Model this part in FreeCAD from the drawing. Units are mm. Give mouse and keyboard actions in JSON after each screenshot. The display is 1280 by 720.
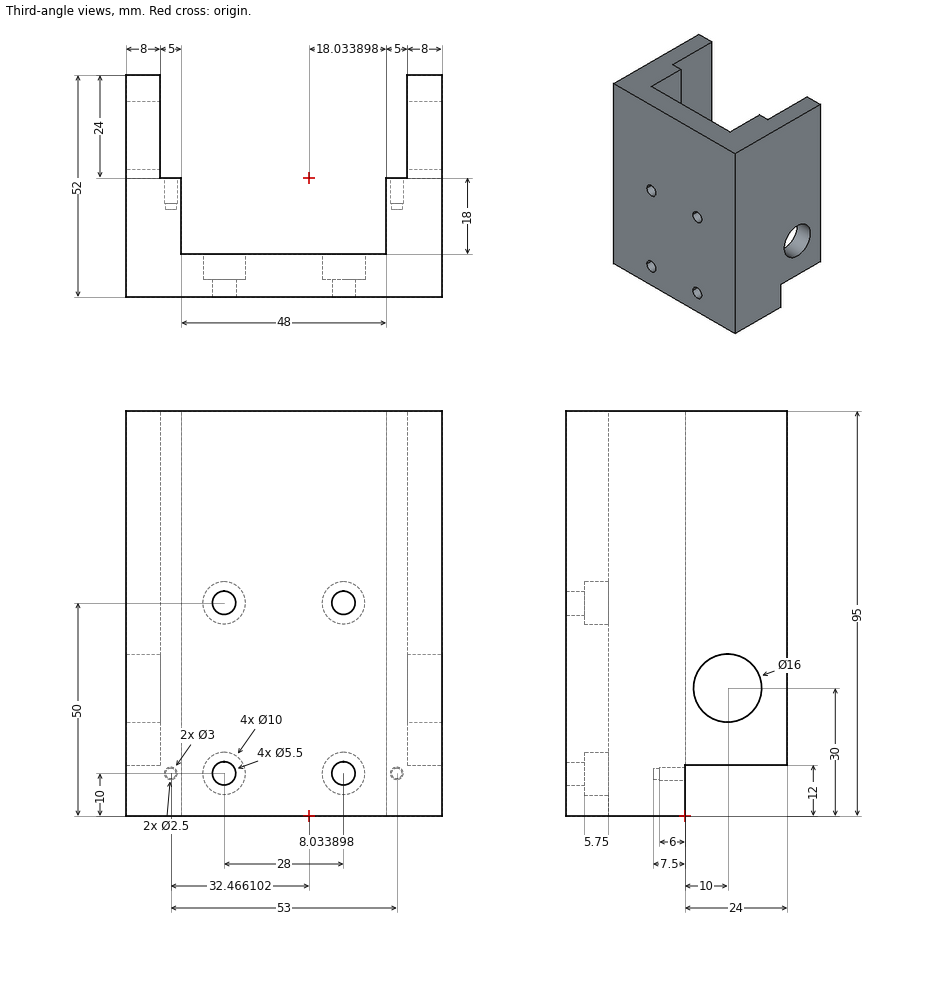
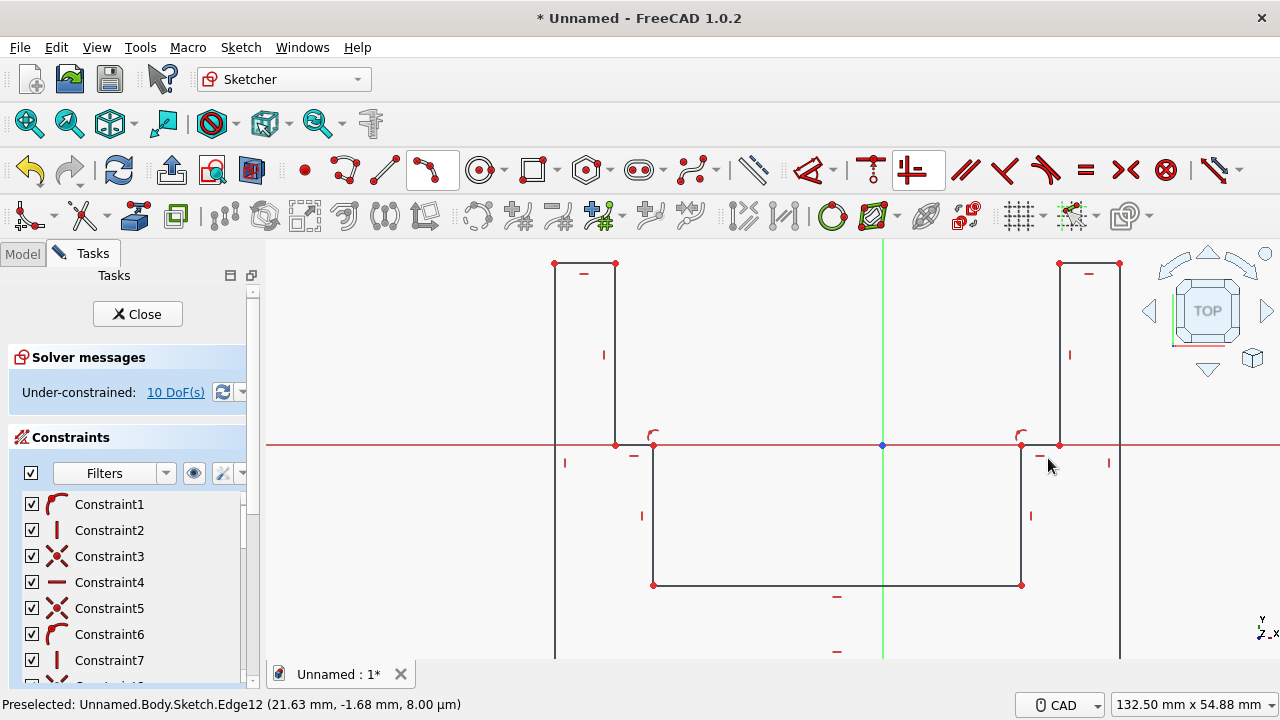
{"action": "left_click", "coordinate": [642, 445]}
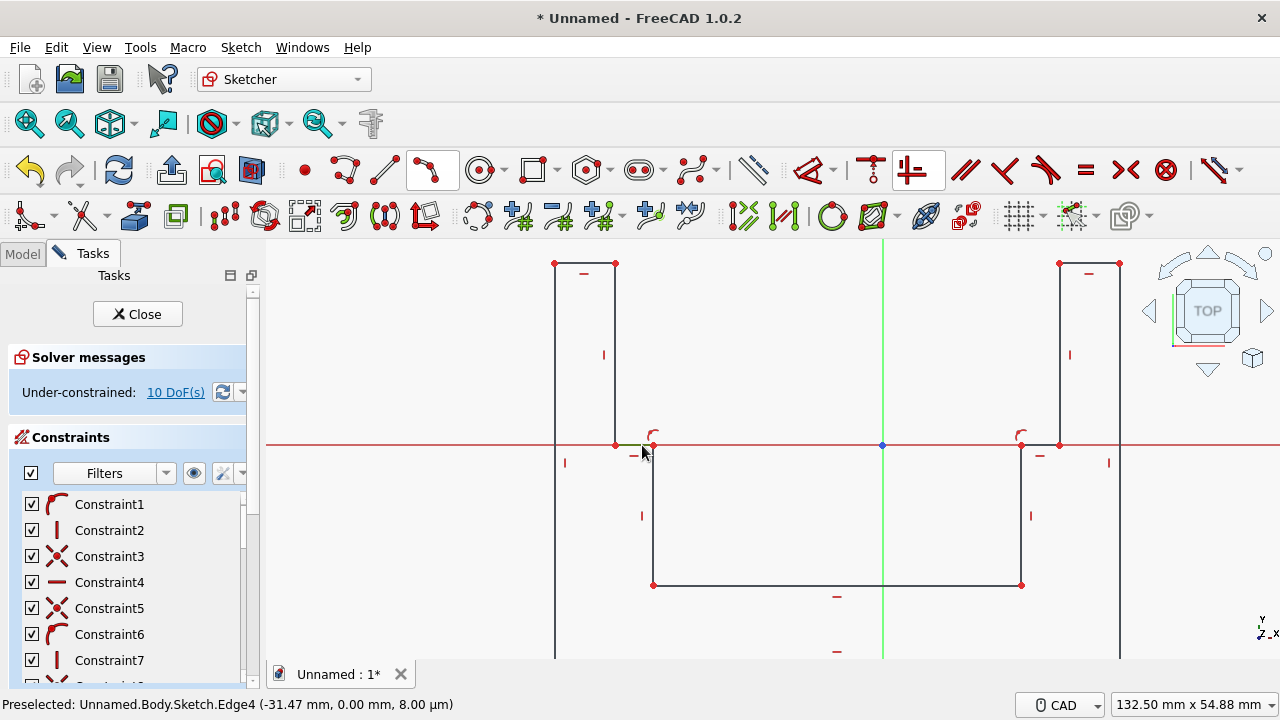
{"action": "left_click", "coordinate": [836, 170]}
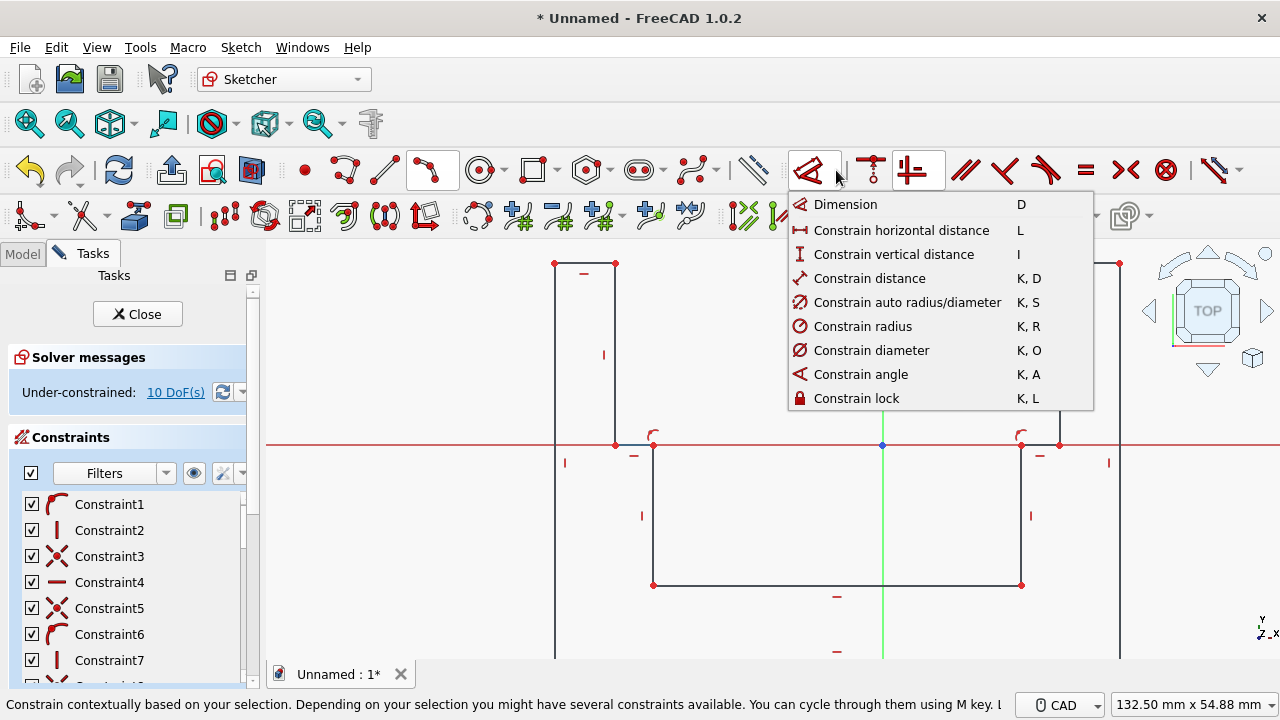
{"action": "left_click", "coordinate": [941, 230]}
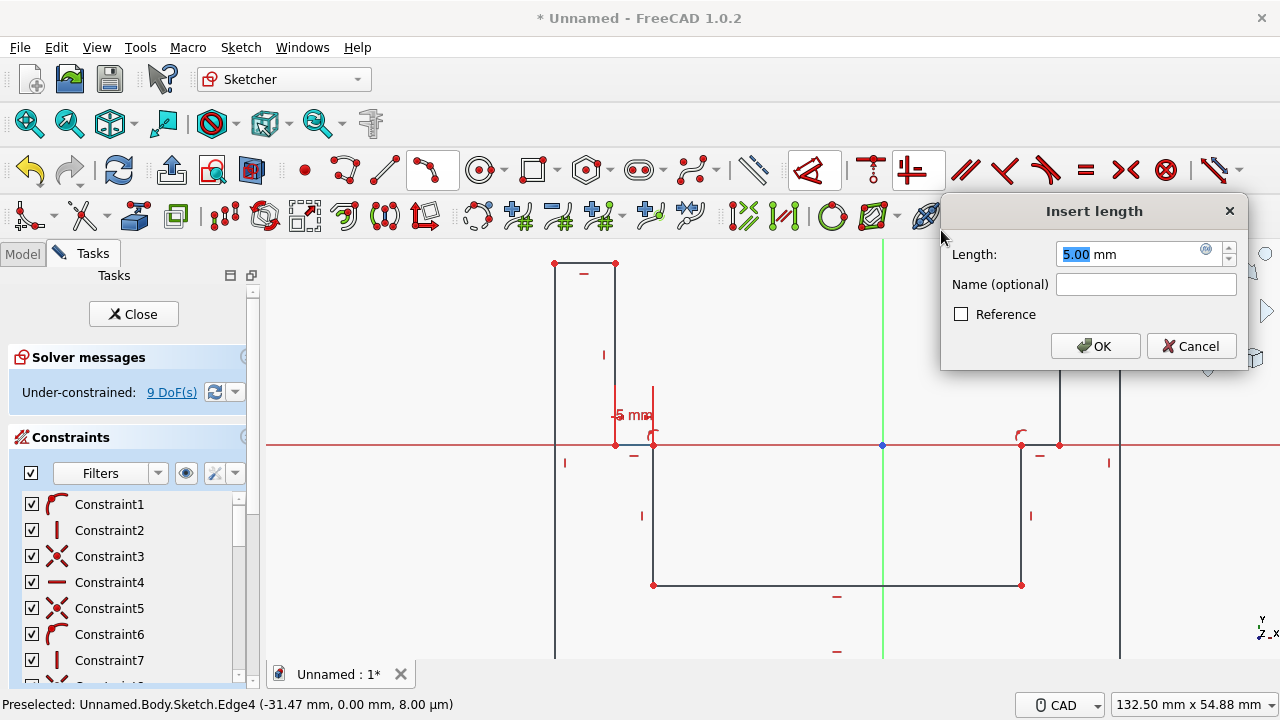
{"action": "type", "text": "5"}
{"action": "key", "text": "Return"}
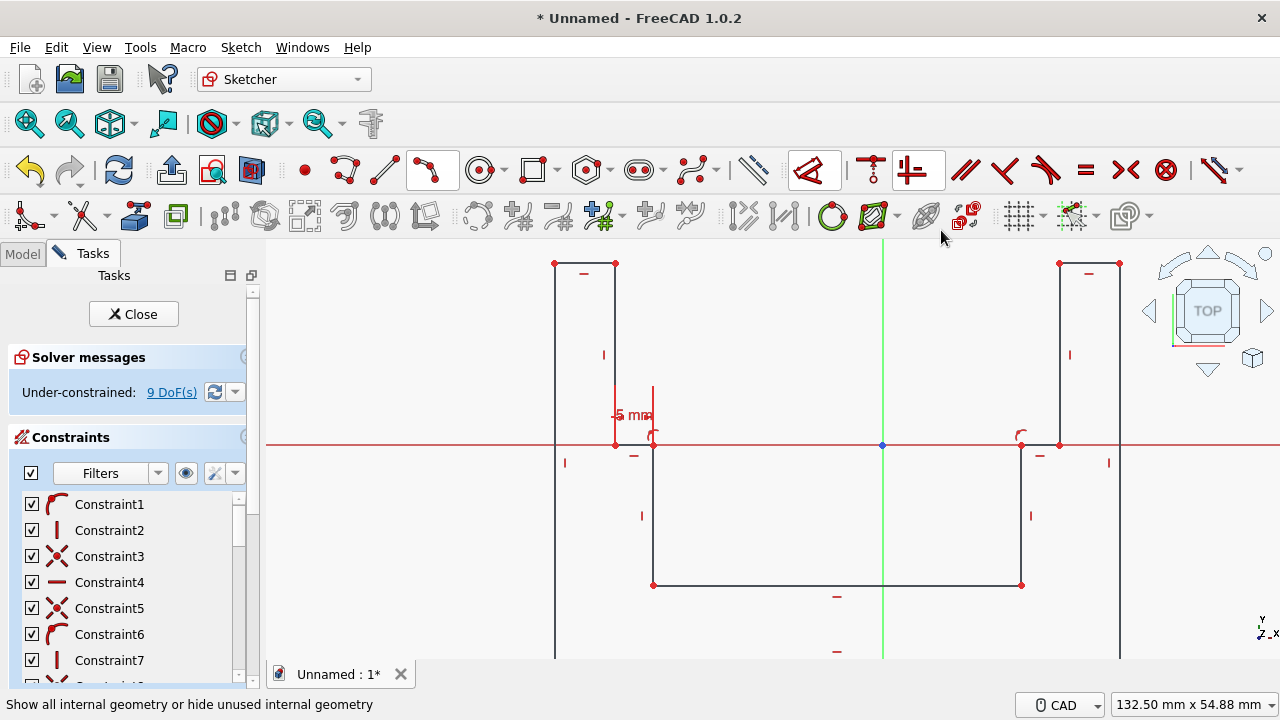
{"action": "scroll", "coordinate": [435, 425], "scroll_direction": "down", "scroll_amount": 2}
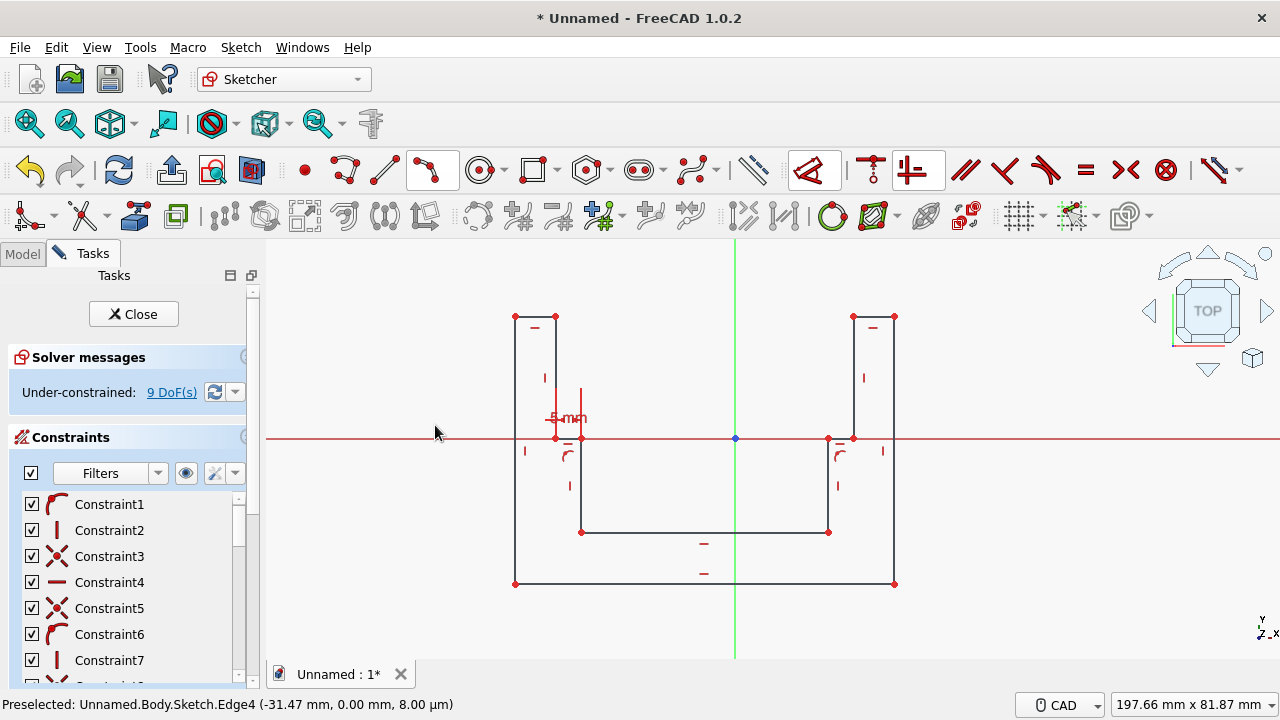
{"action": "left_click", "coordinate": [544, 317]}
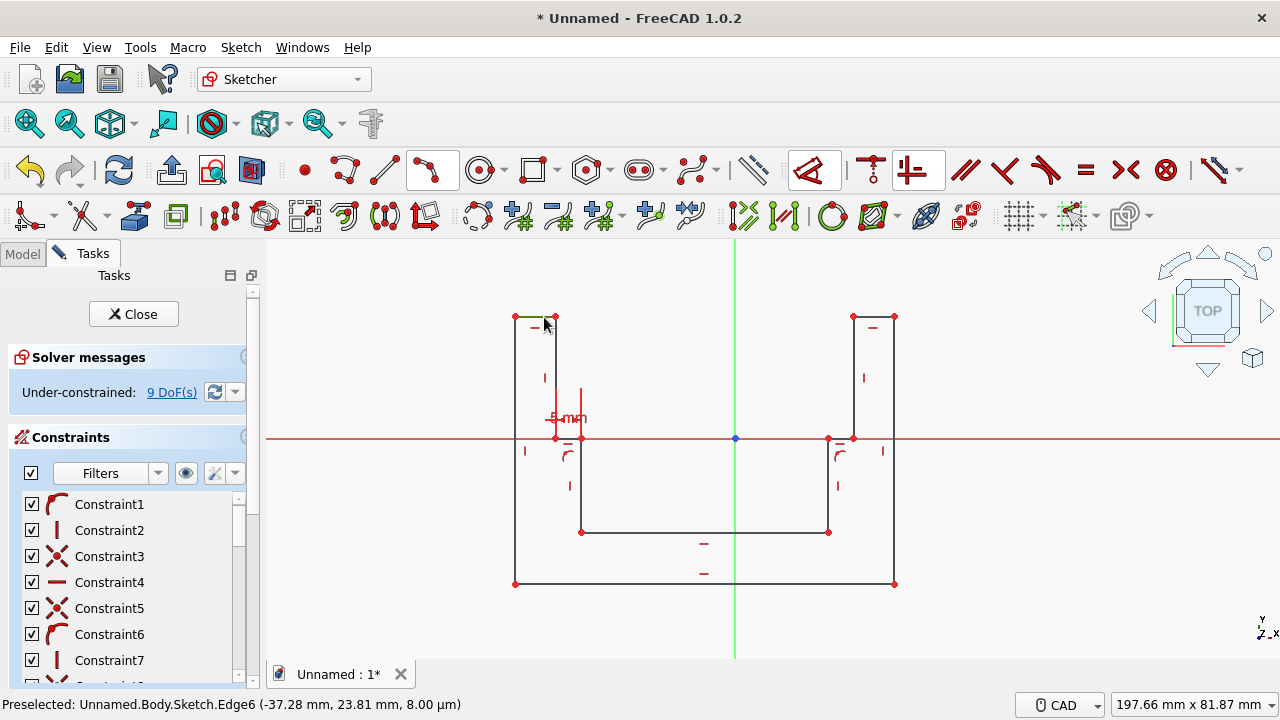
{"action": "key", "text": "l"}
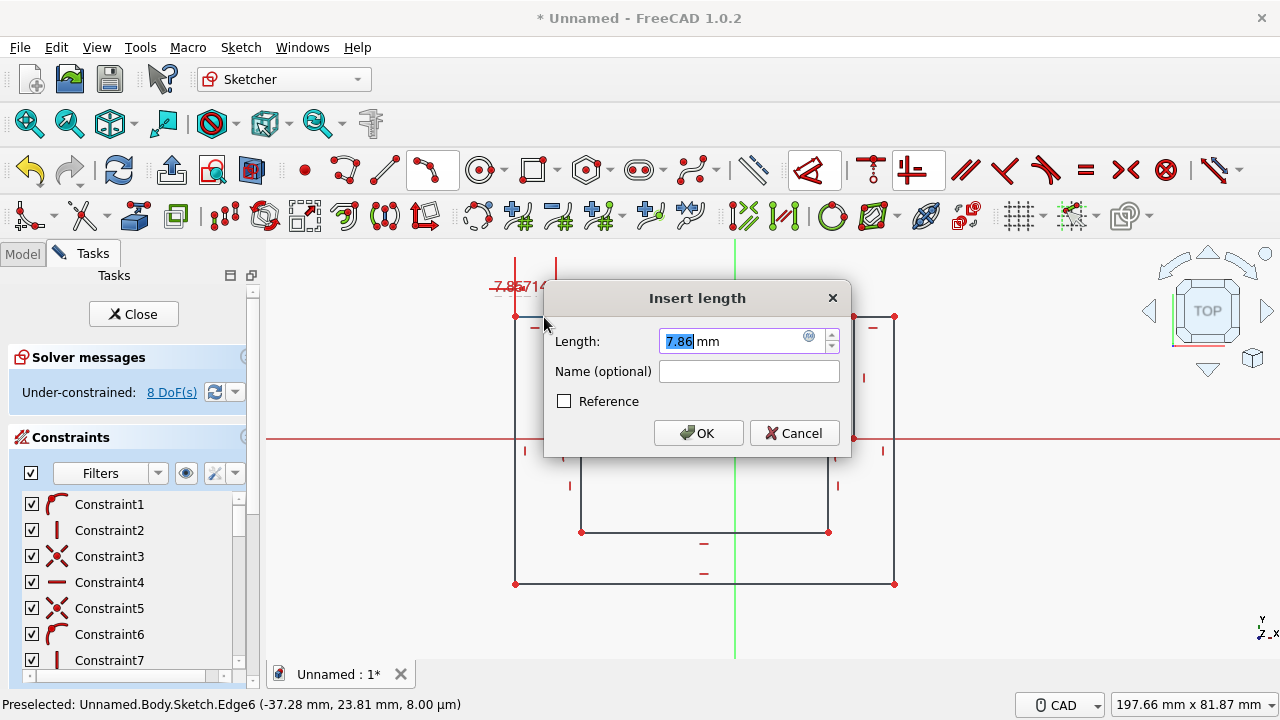
{"action": "type", "text": "8"}
{"action": "key", "text": "Return"}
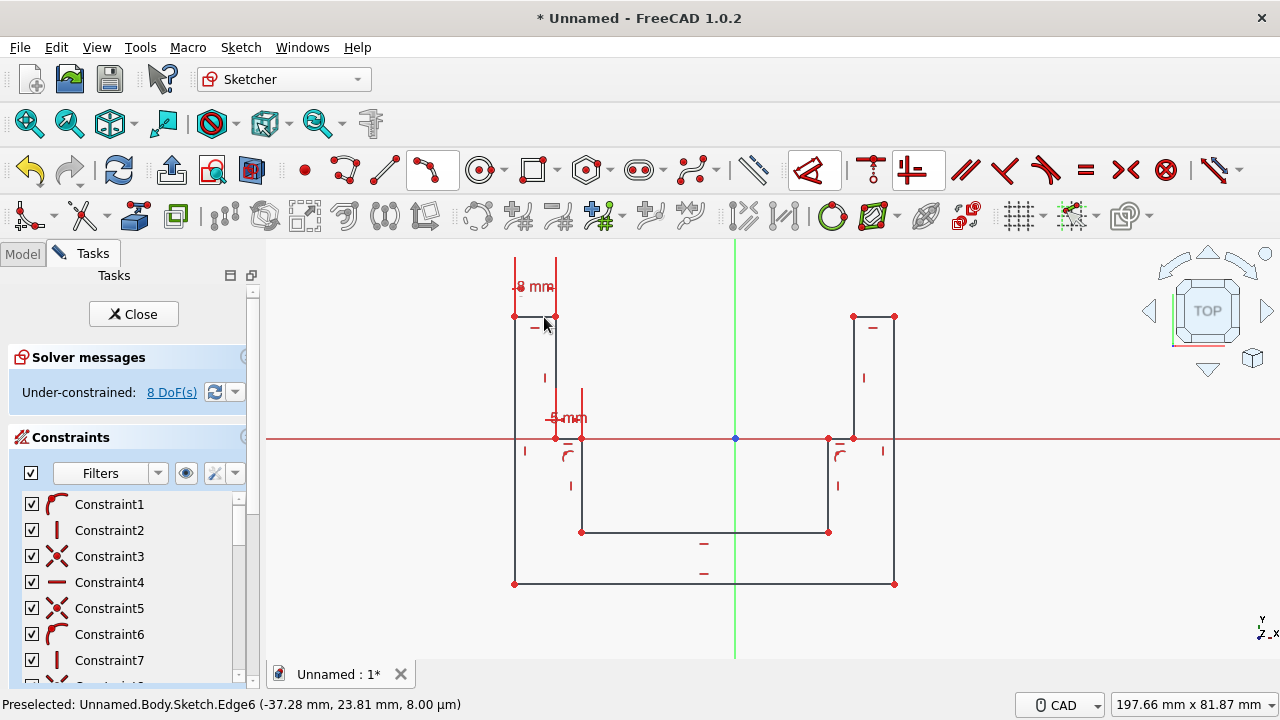
{"action": "left_click", "coordinate": [882, 317]}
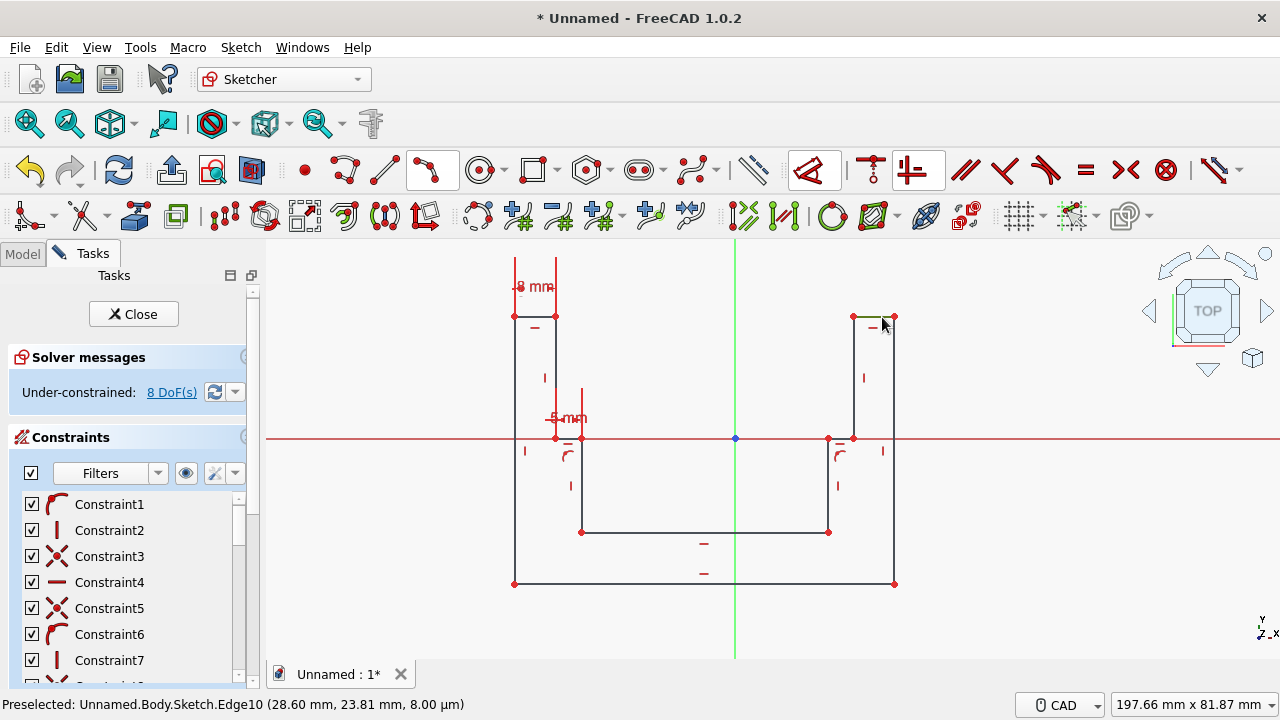
{"action": "key", "text": "l"}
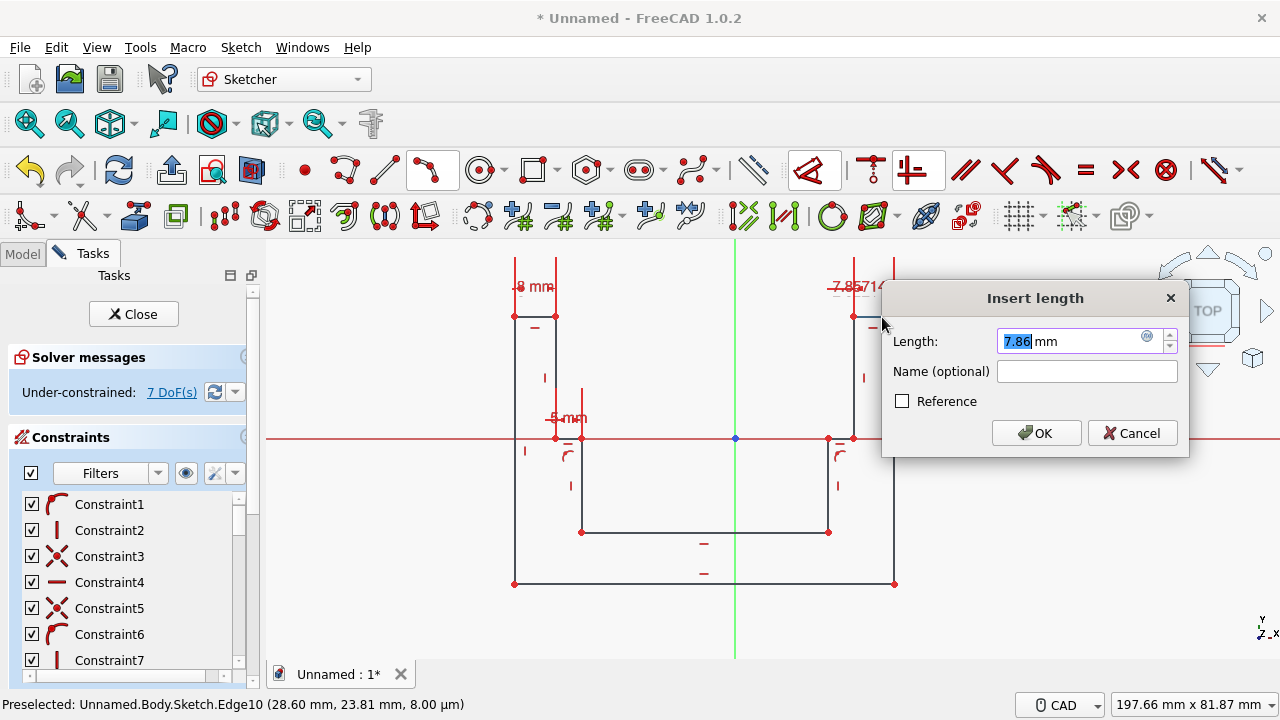
{"action": "type", "text": "8"}
{"action": "key", "text": "Return"}